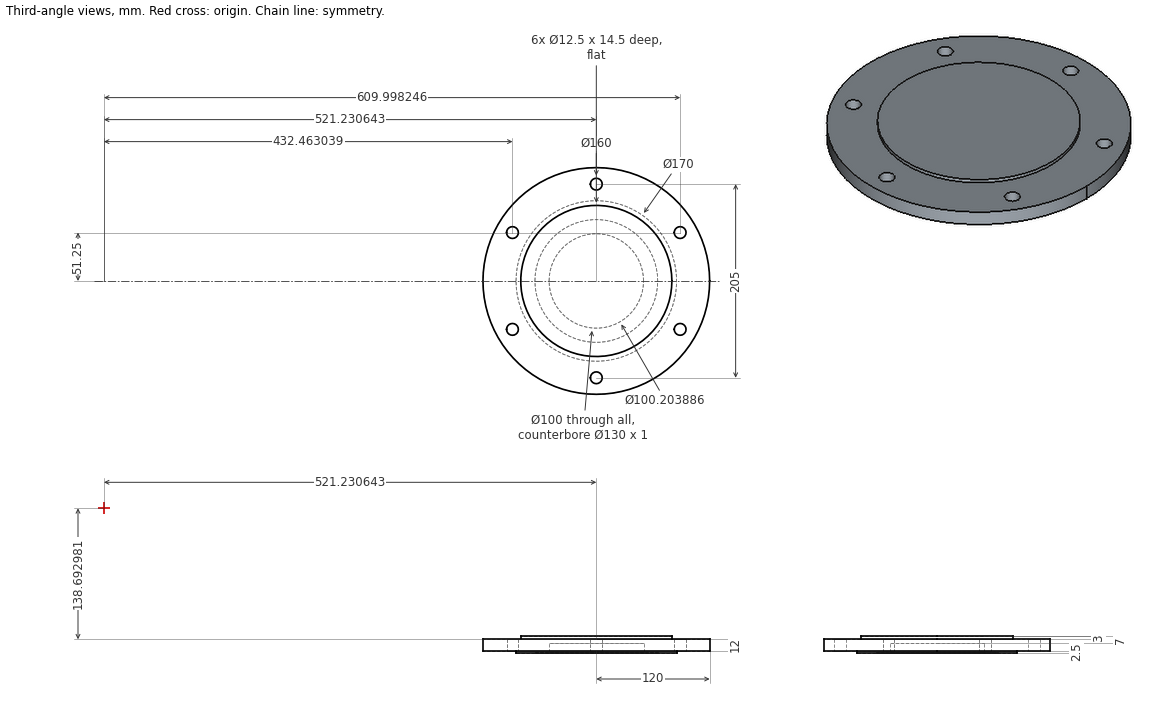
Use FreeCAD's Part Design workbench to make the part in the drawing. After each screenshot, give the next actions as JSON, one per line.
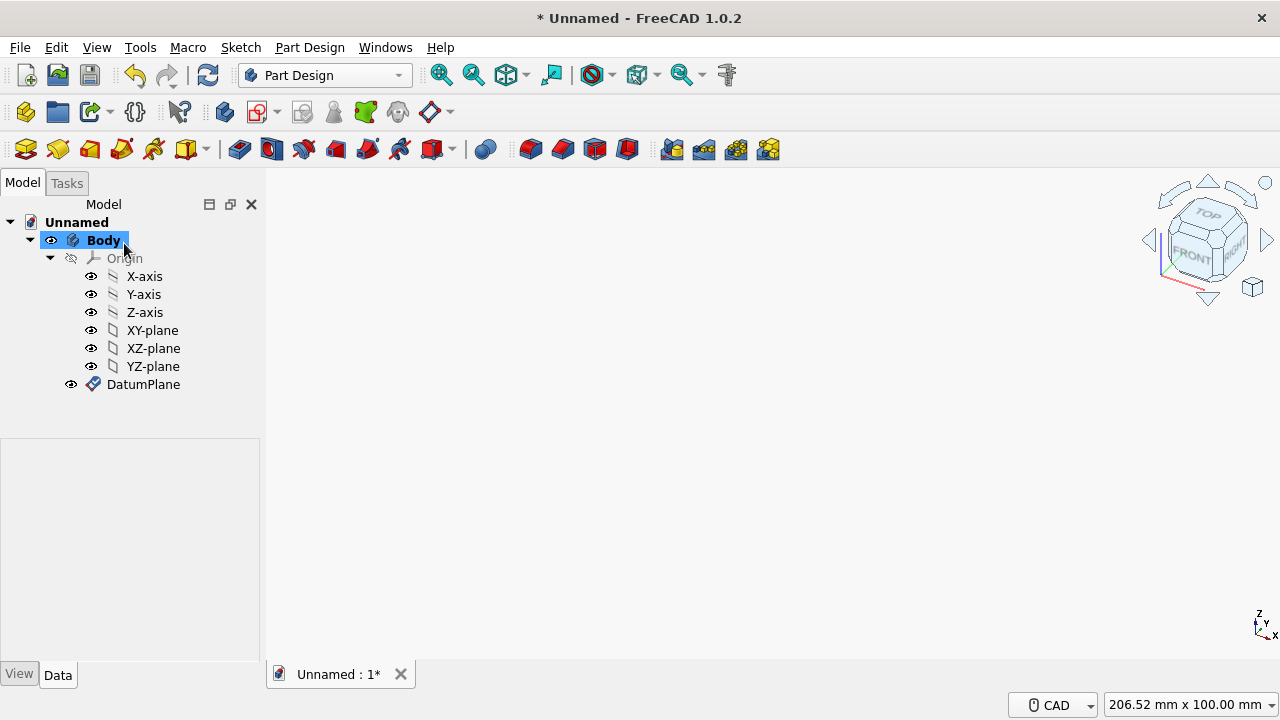
{"action": "left_click", "coordinate": [116, 384]}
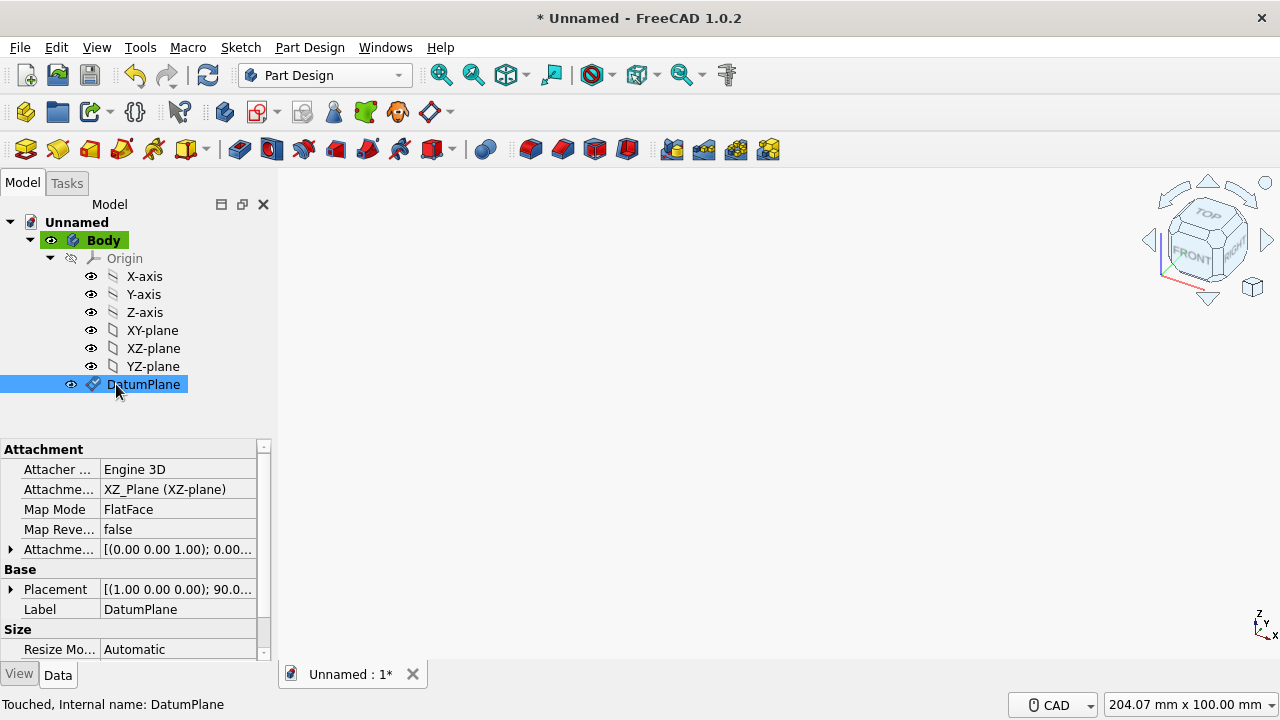
{"action": "left_click", "coordinate": [258, 112]}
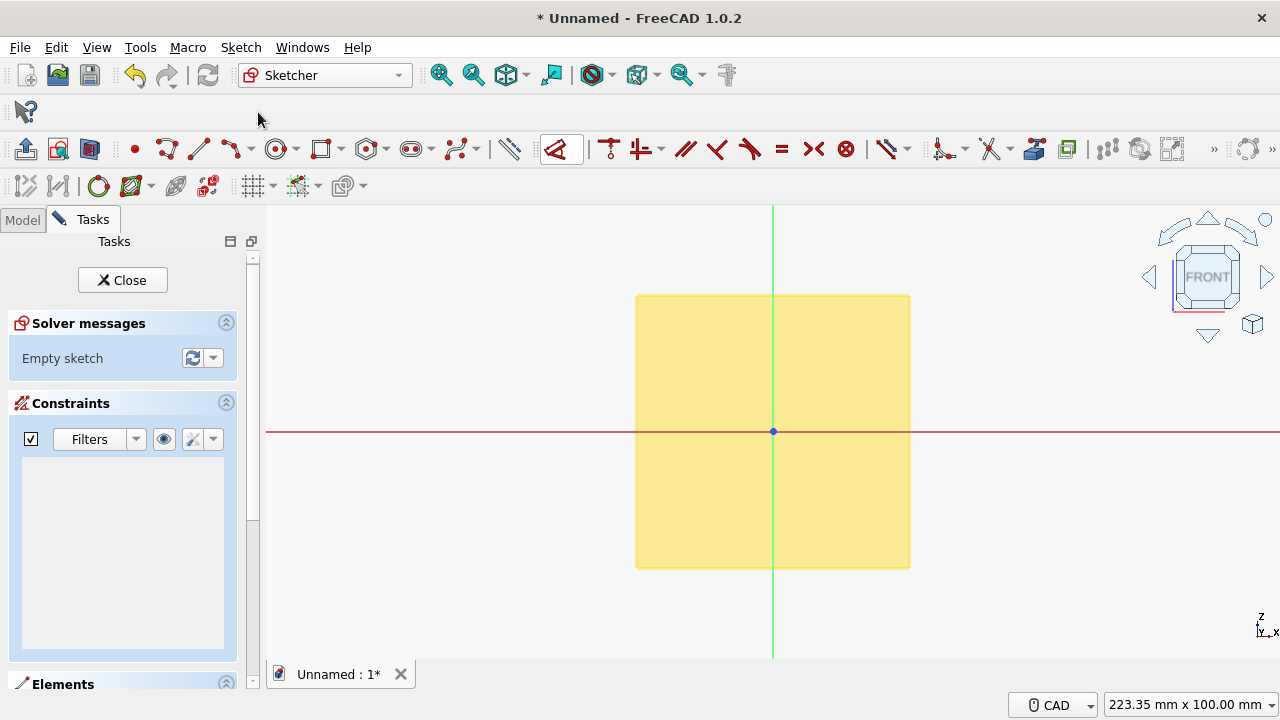
{"action": "scroll", "coordinate": [704, 432], "scroll_direction": "down", "scroll_amount": 5}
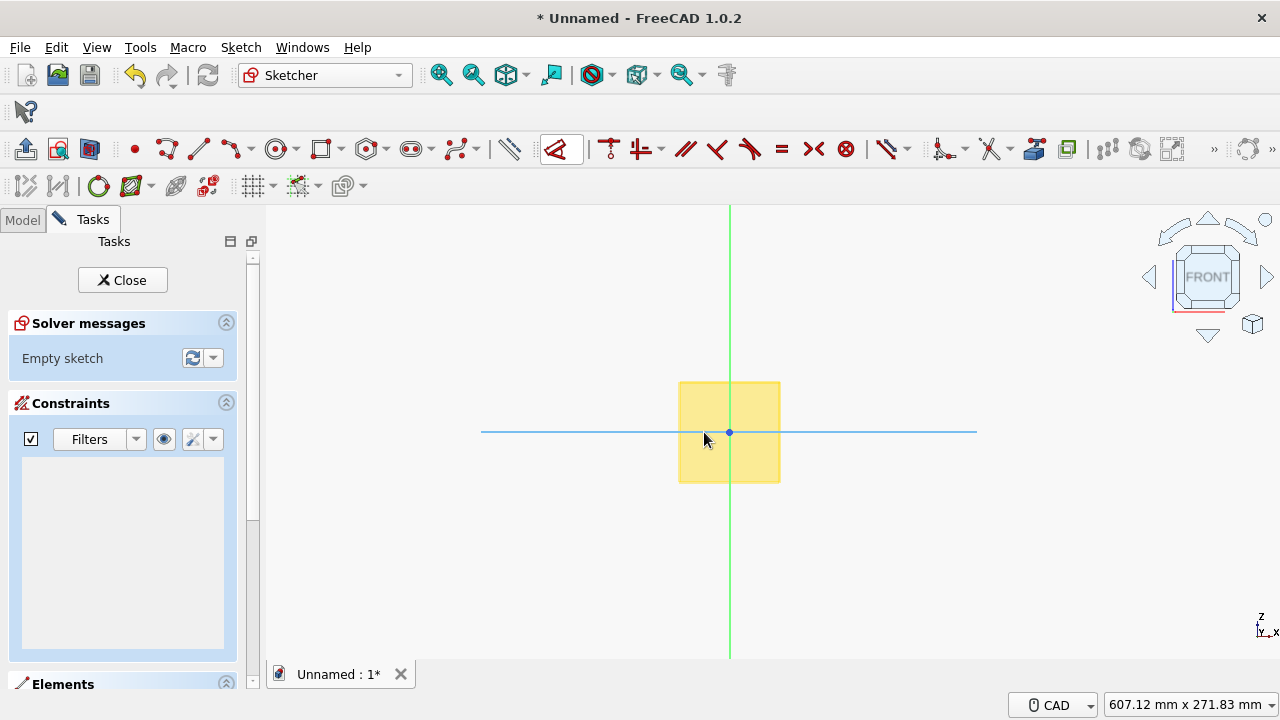
{"action": "scroll", "coordinate": [704, 432], "scroll_direction": "down", "scroll_amount": 5}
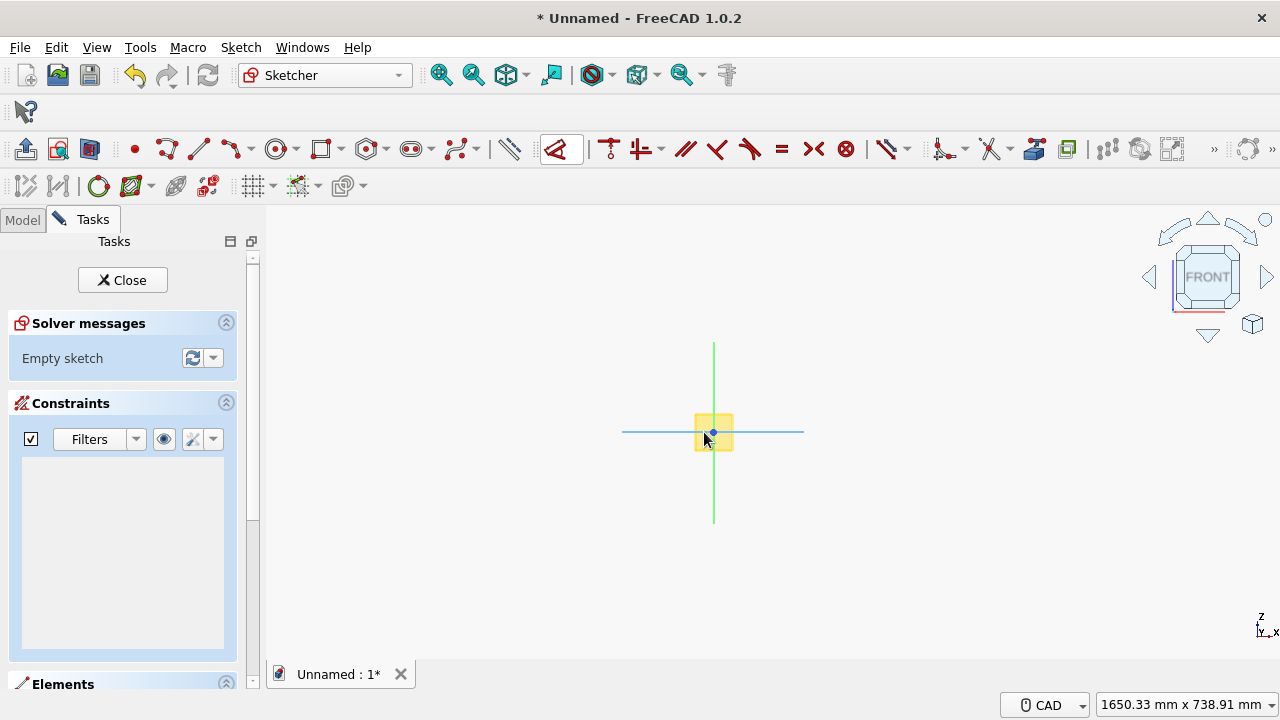
{"action": "scroll", "coordinate": [1115, 528], "scroll_direction": "up", "scroll_amount": 10}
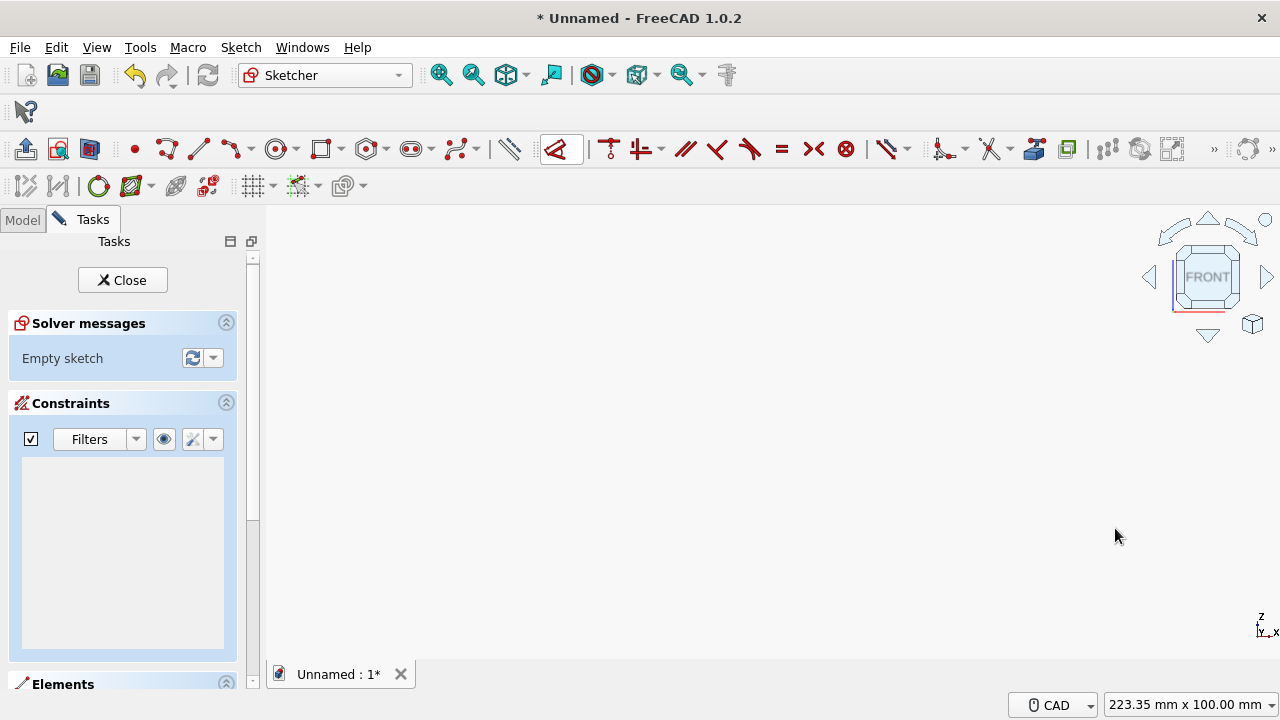
{"action": "key", "text": "g r"}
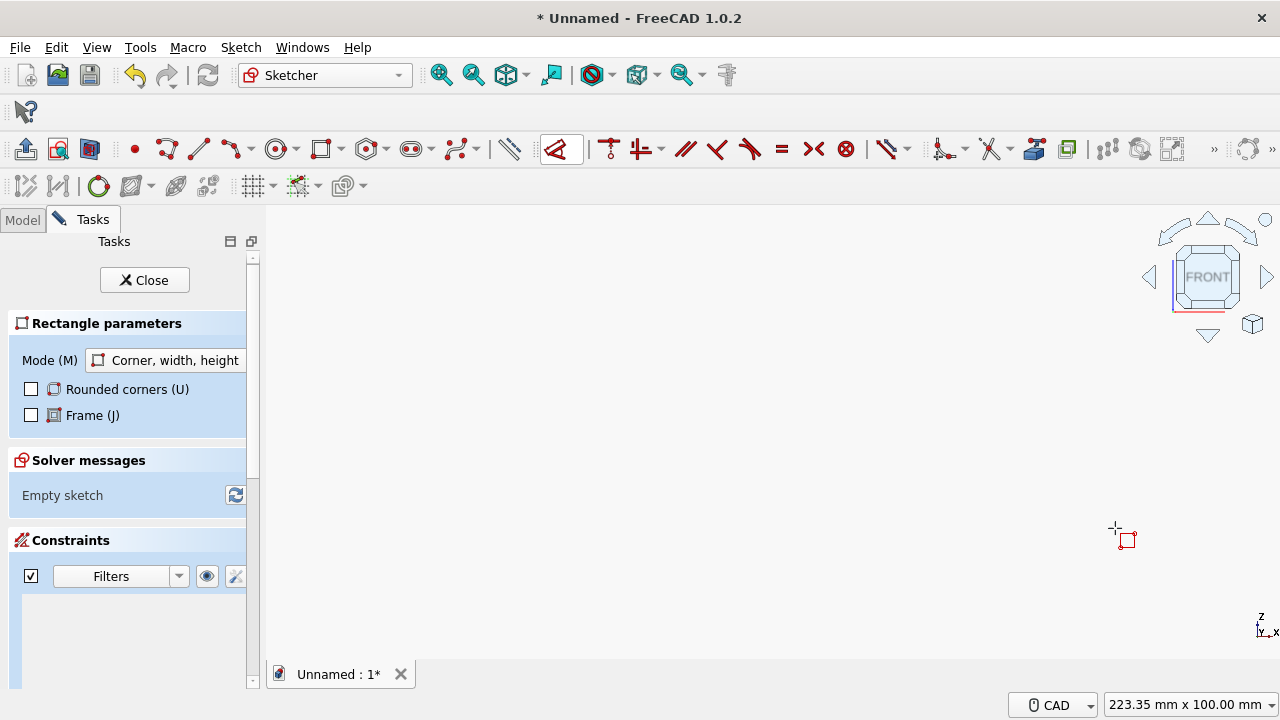
{"action": "left_click", "coordinate": [511, 447]}
{"action": "mouse_move", "coordinate": [1056, 501]}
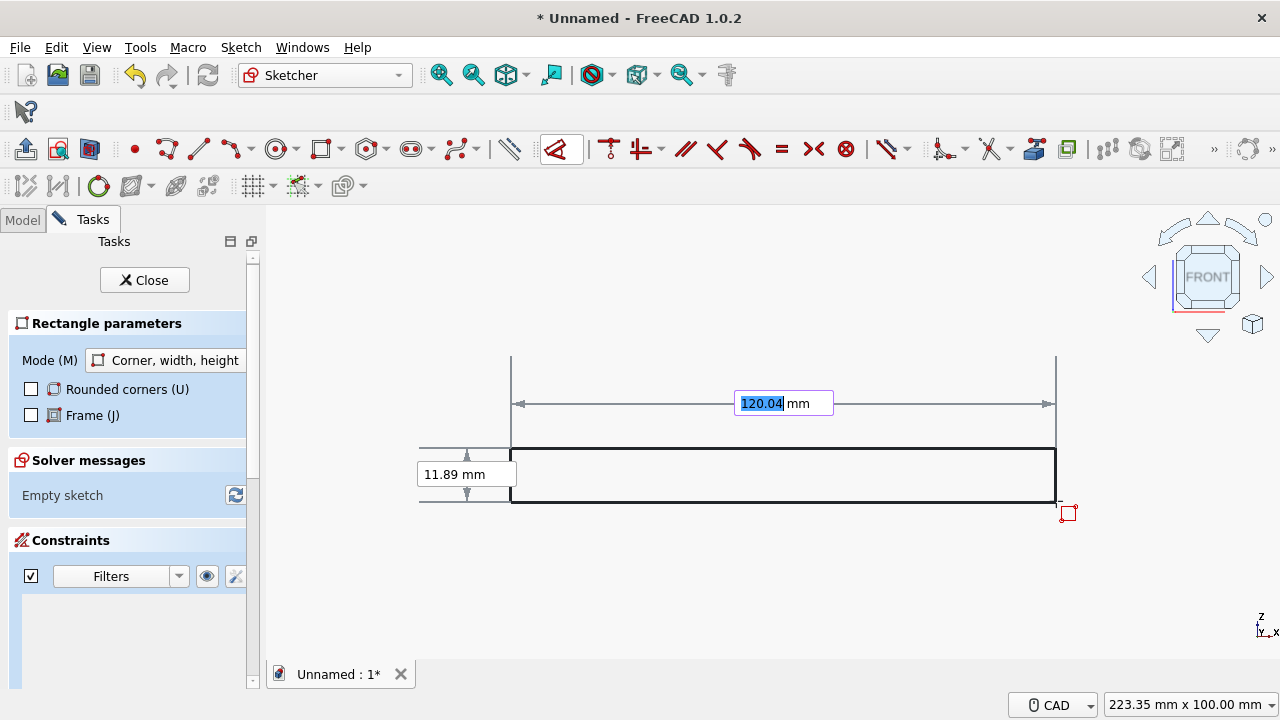
{"action": "type", "text": "120"}
{"action": "key", "text": "Tab"}
{"action": "type", "text": "12"}
{"action": "key", "text": "Return"}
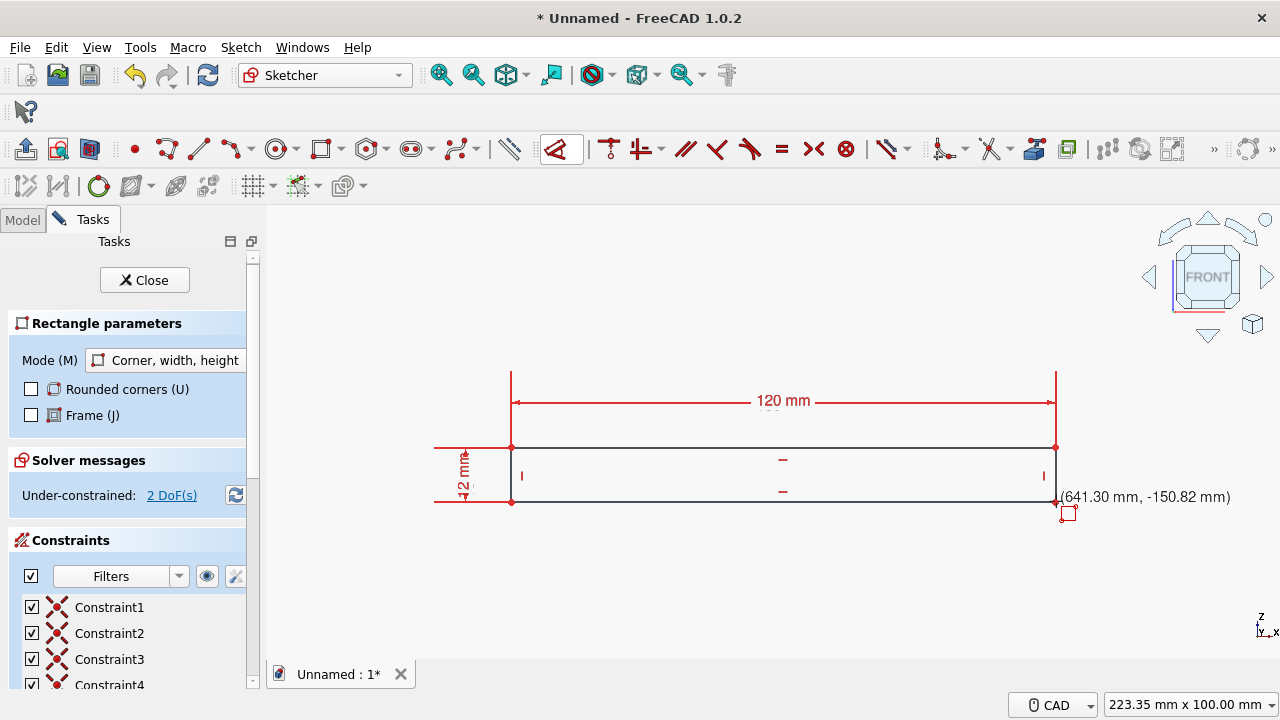
{"action": "key", "text": "g l"}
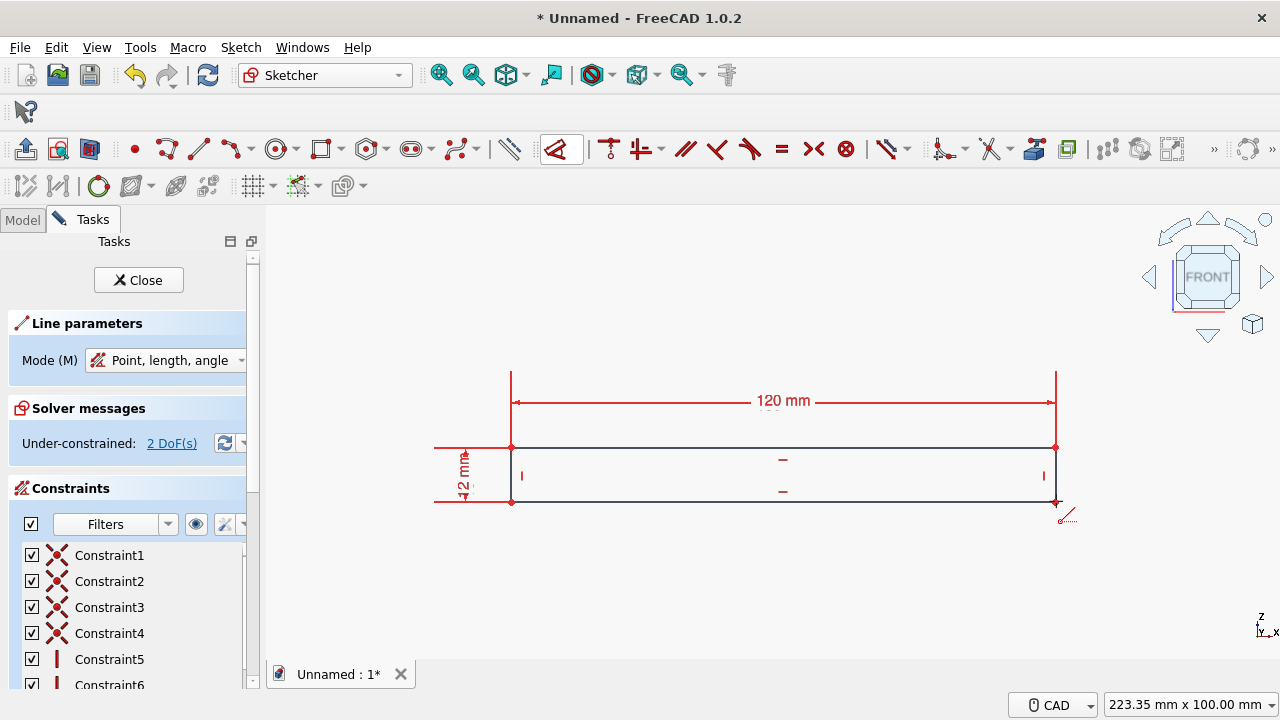
{"action": "left_click", "coordinate": [511, 425]}
{"action": "left_click", "coordinate": [511, 360]}
{"action": "key", "text": "Escape"}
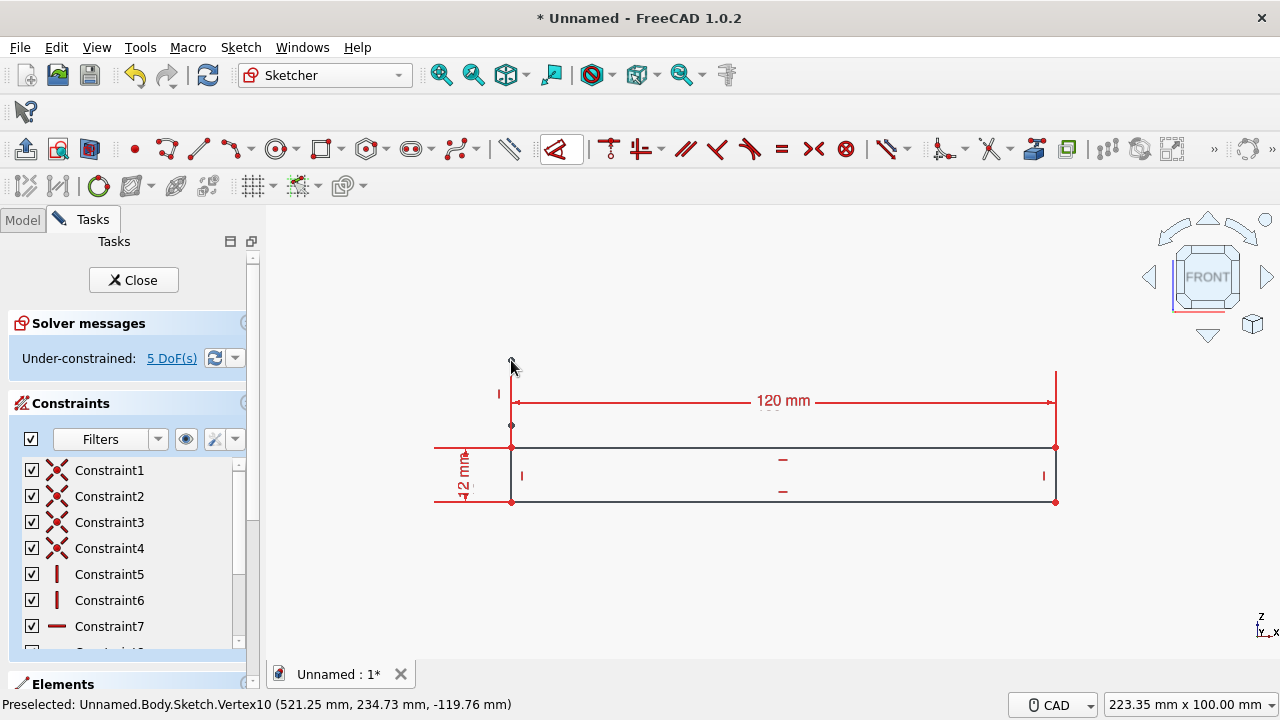
{"action": "left_click", "coordinate": [511, 407]}